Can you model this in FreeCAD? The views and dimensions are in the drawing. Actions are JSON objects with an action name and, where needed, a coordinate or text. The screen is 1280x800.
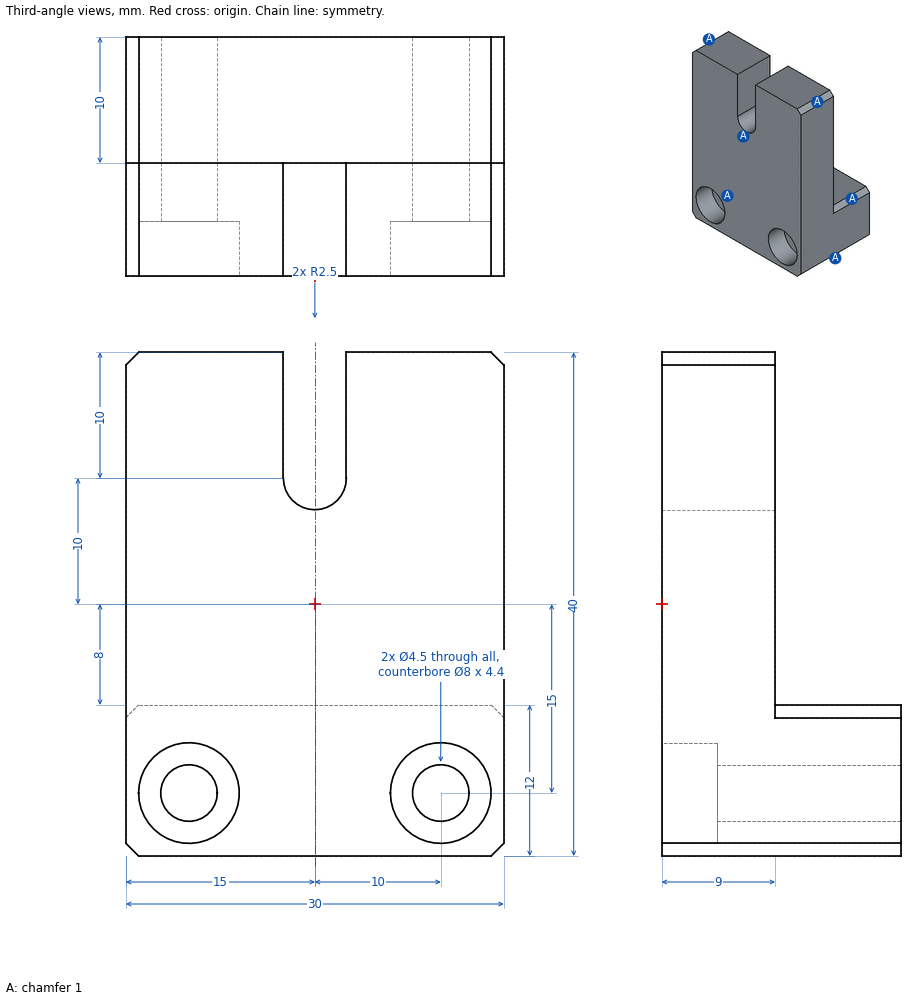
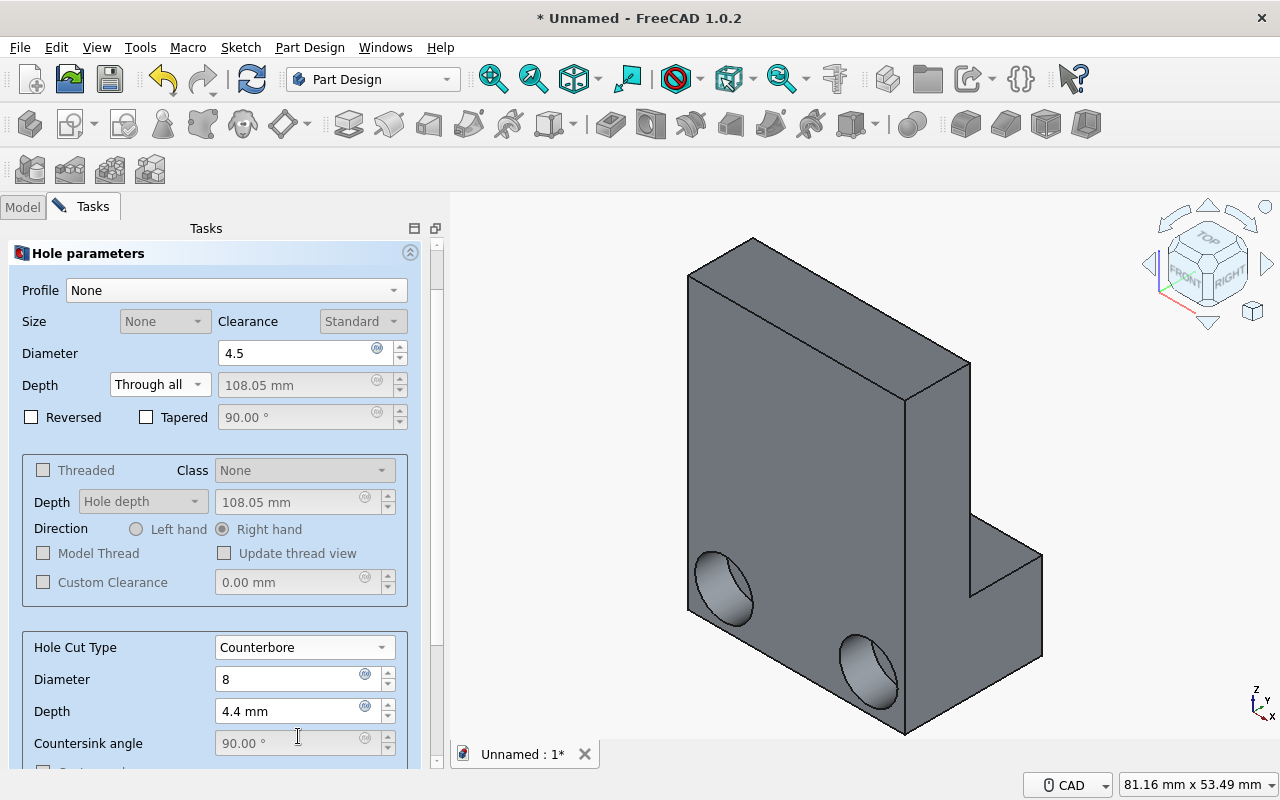
{"action": "scroll", "coordinate": [437, 503], "scroll_direction": "up", "scroll_amount": 2}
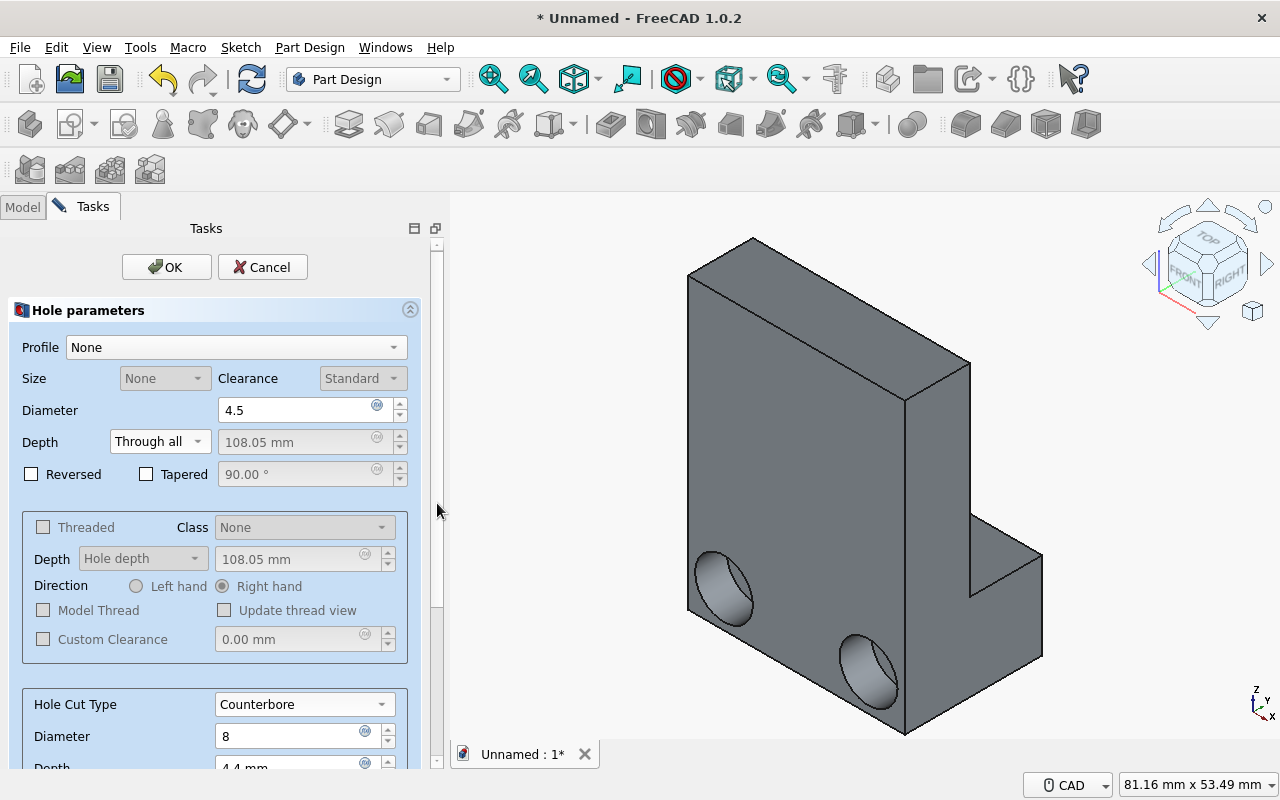
{"action": "left_click", "coordinate": [167, 267]}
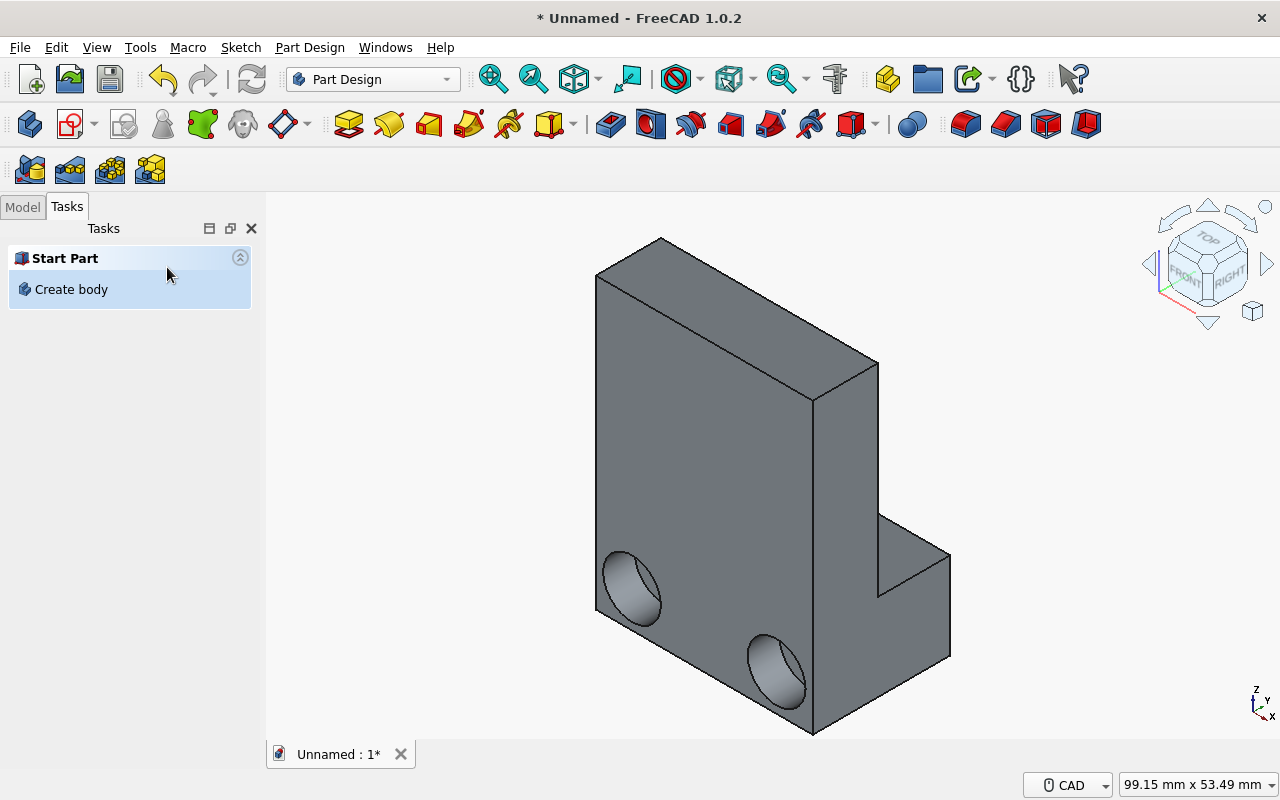
{"action": "left_click", "coordinate": [914, 575]}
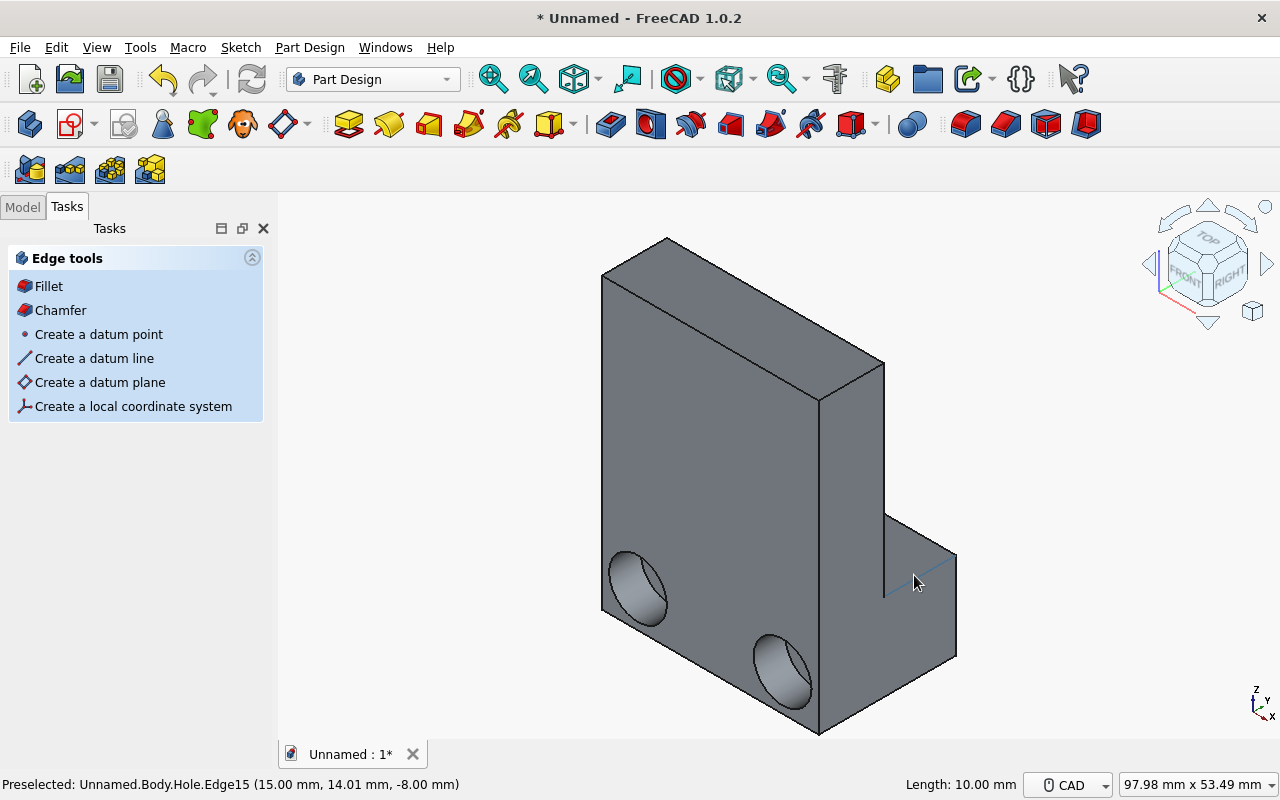
{"action": "left_click", "coordinate": [851, 381], "text": "ctrl"}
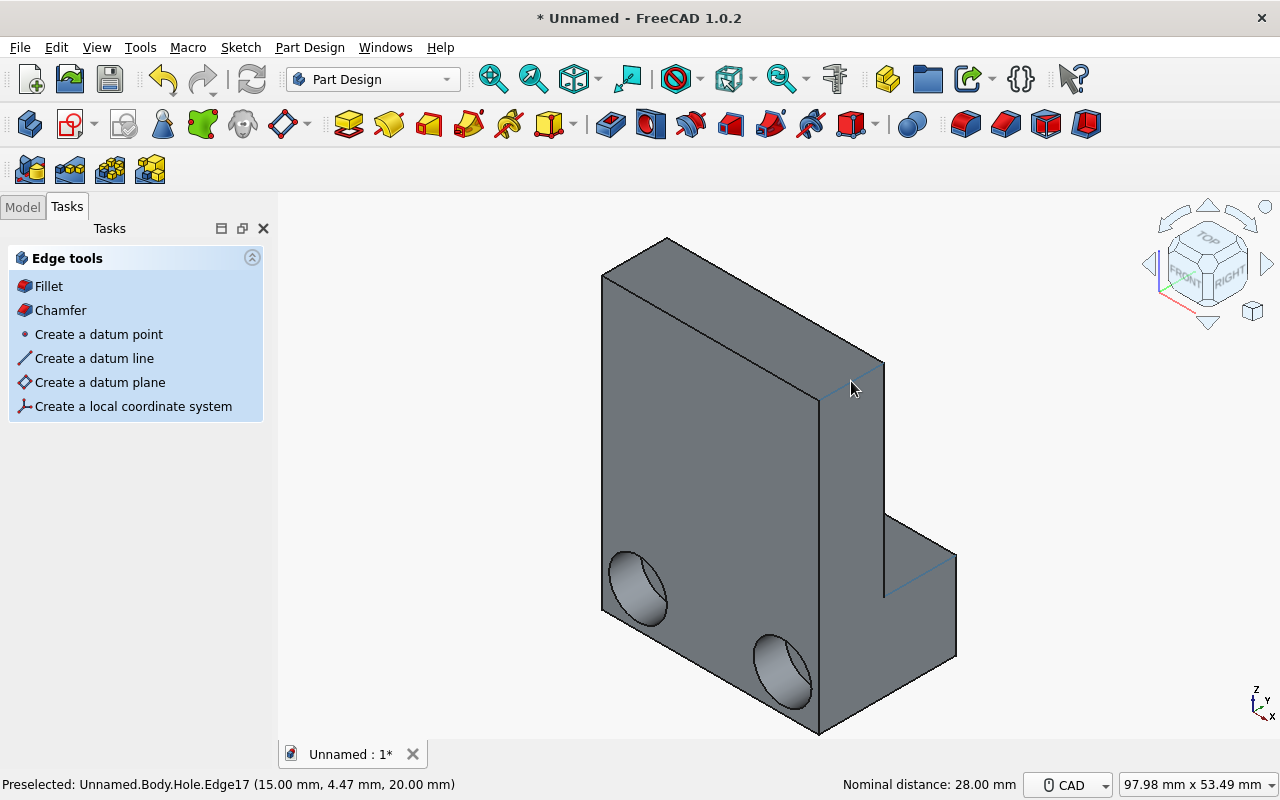
{"action": "key", "text": "2"}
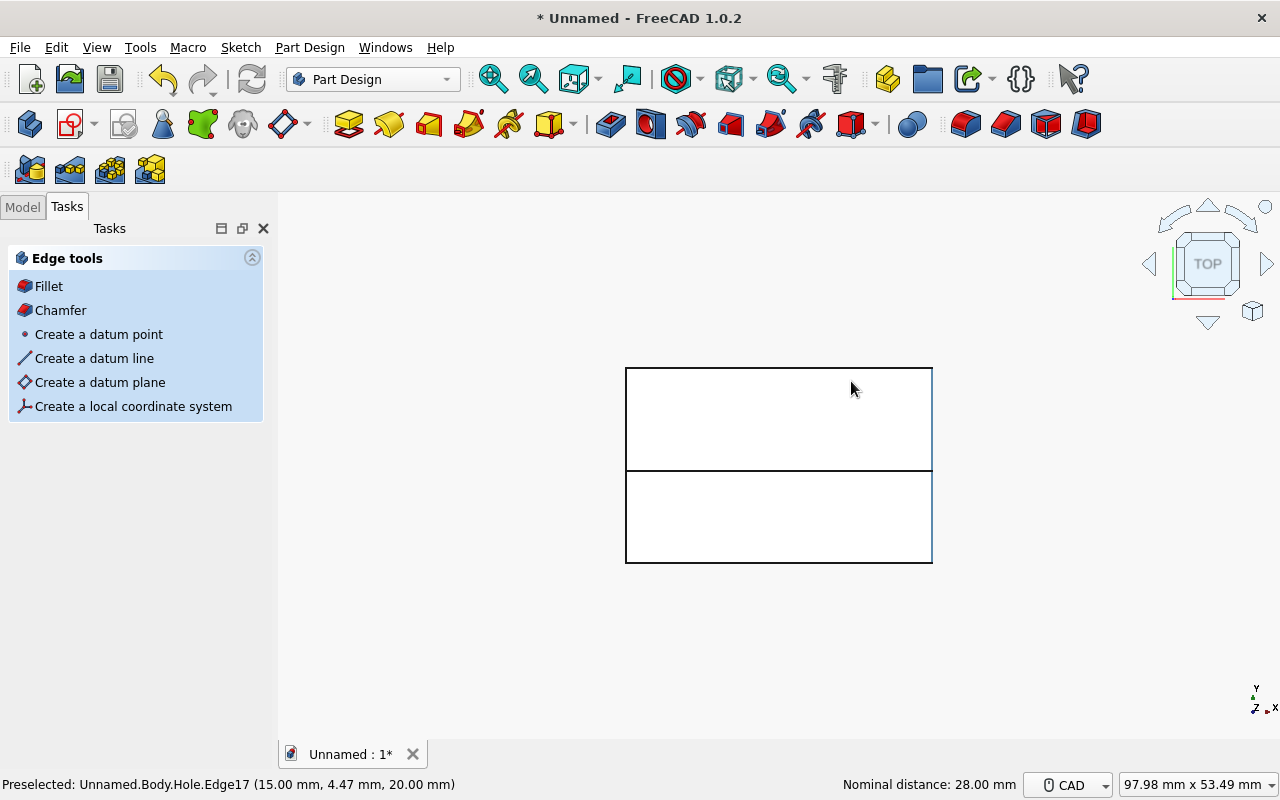
{"action": "left_click", "coordinate": [494, 80]}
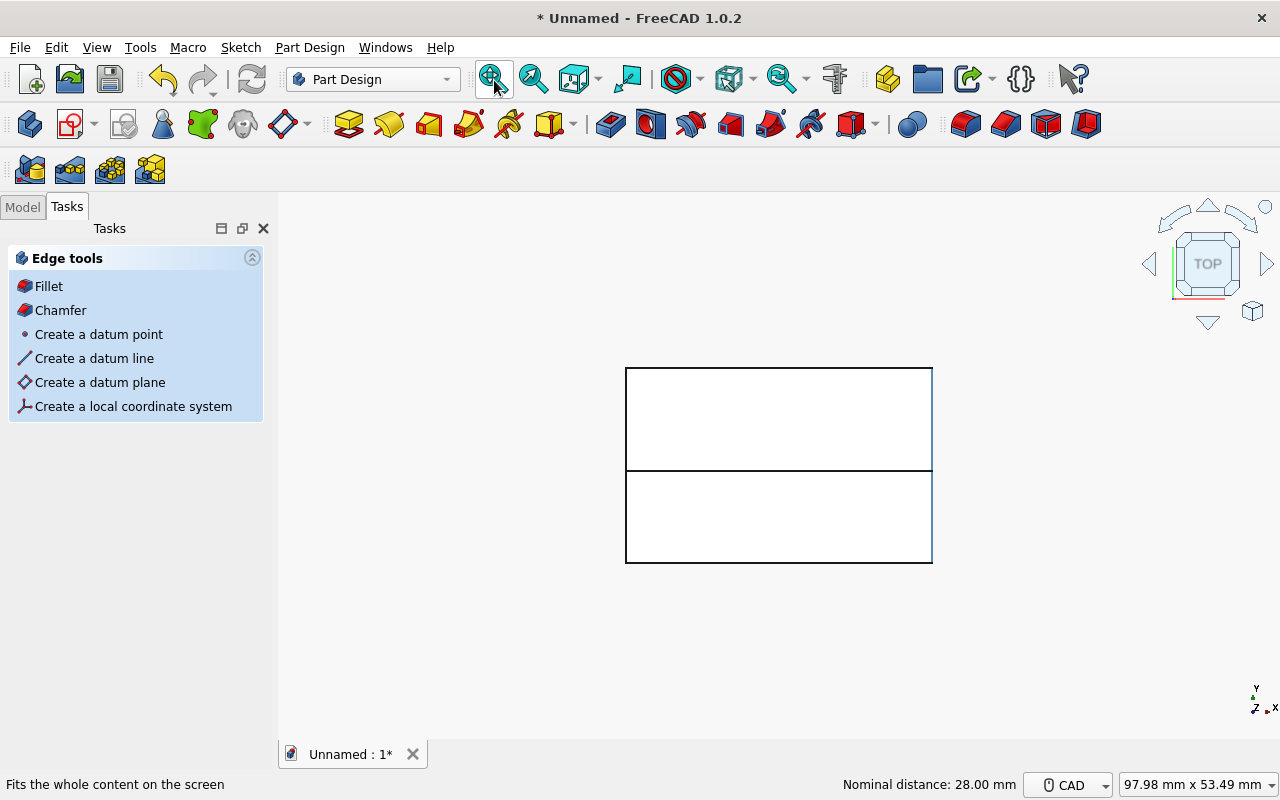
{"action": "left_click", "coordinate": [626, 418], "text": "ctrl"}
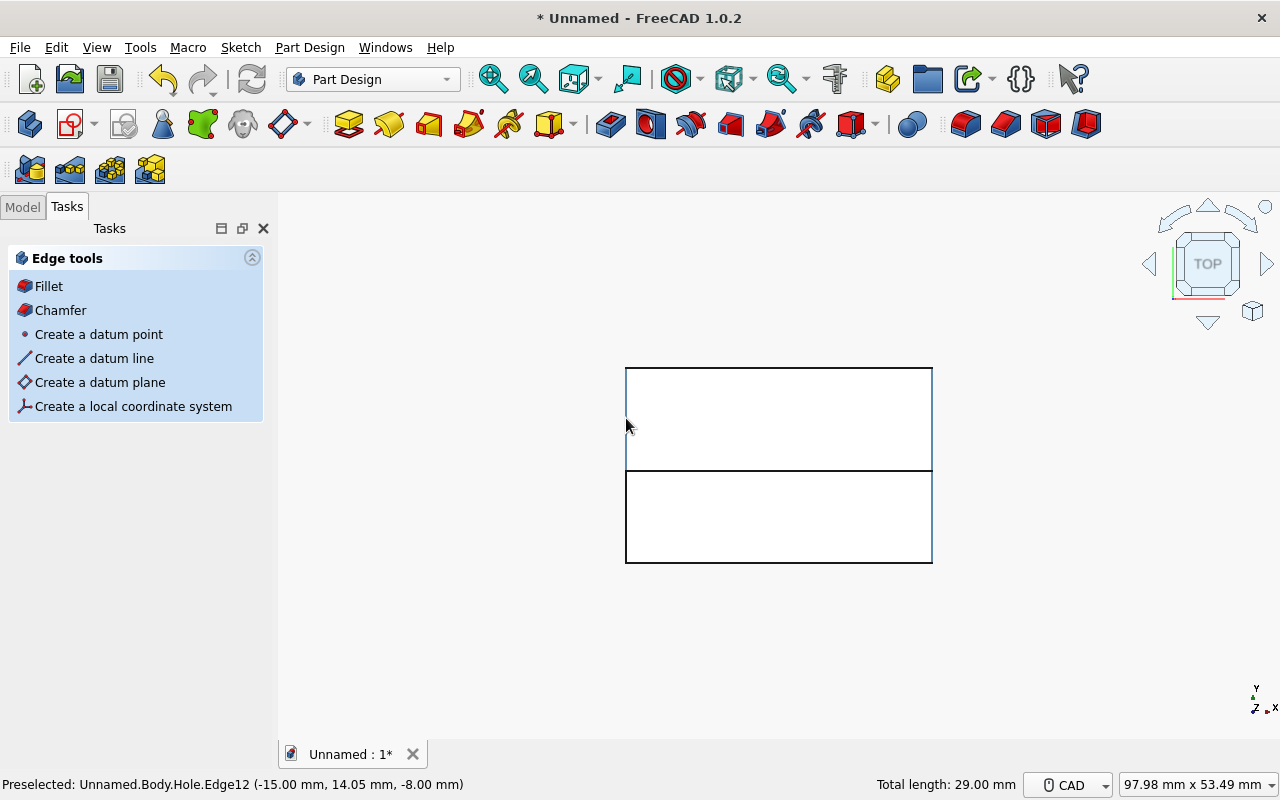
{"action": "left_click", "coordinate": [626, 516], "text": "ctrl"}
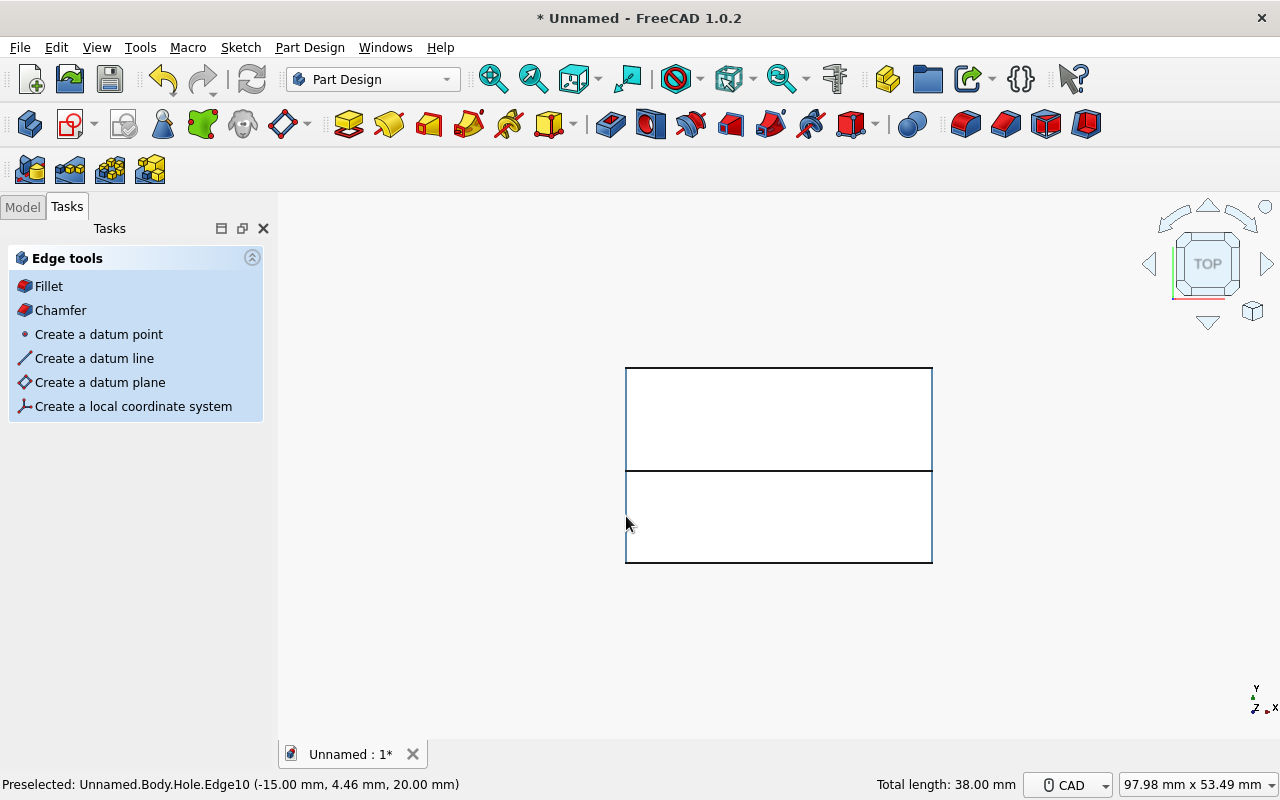
{"action": "key", "text": "0"}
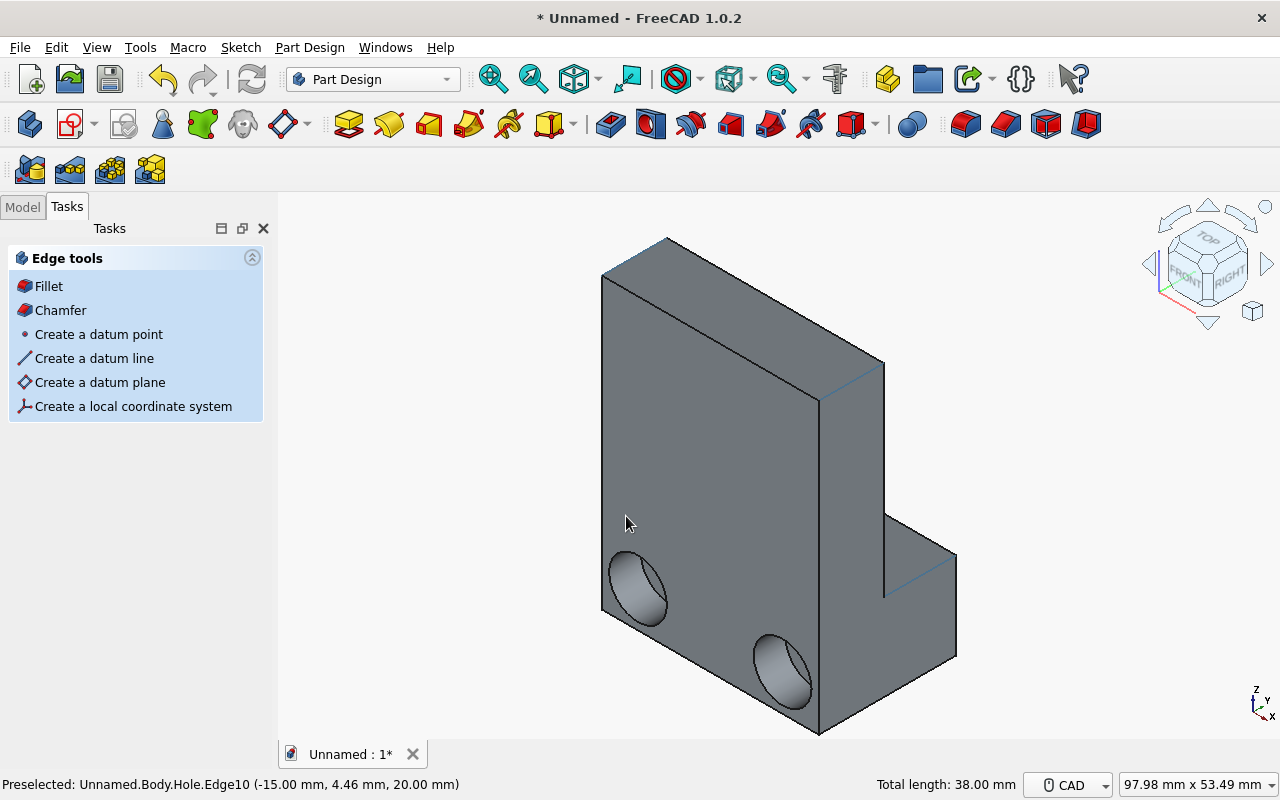
{"action": "key", "text": "1"}